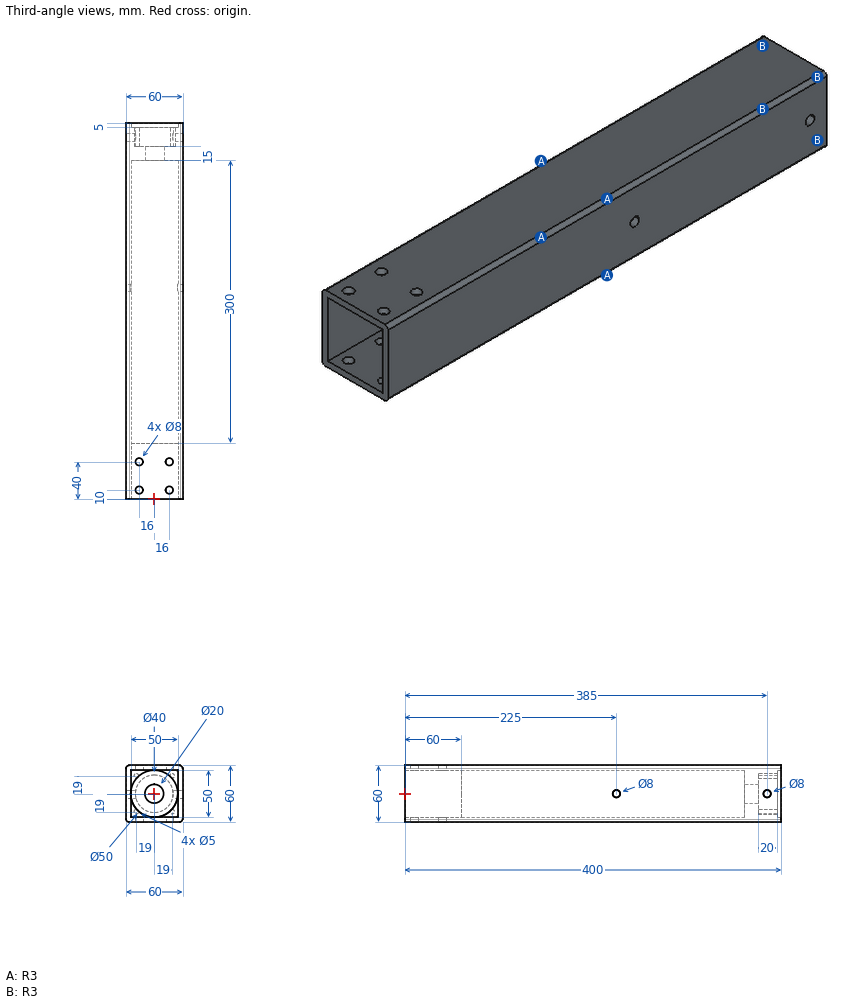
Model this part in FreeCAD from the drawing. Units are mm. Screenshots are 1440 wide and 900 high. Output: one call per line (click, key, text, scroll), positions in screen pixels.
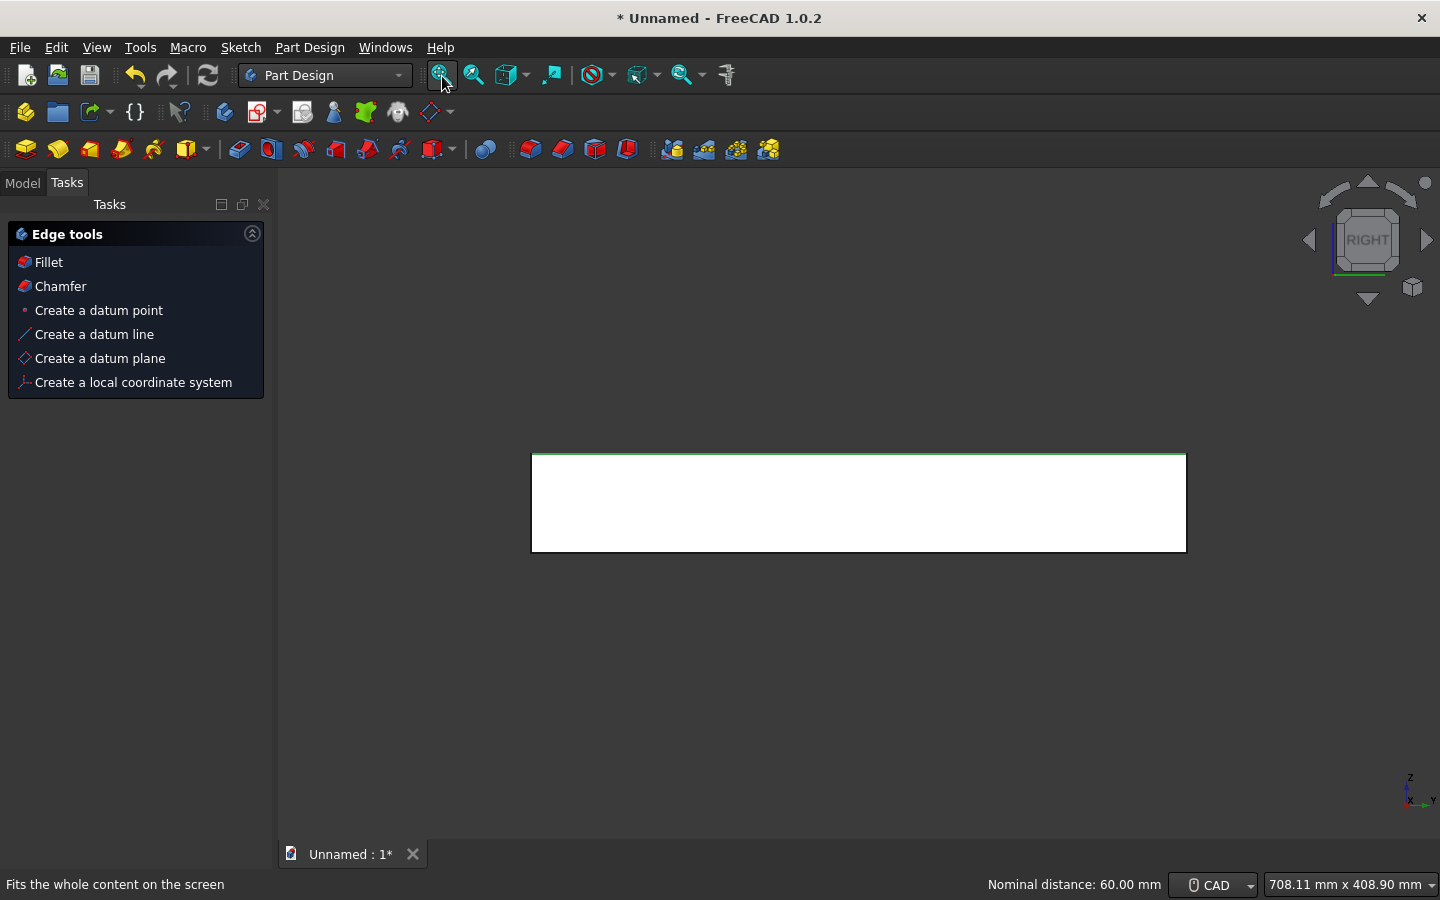
click(859, 552, ctrl)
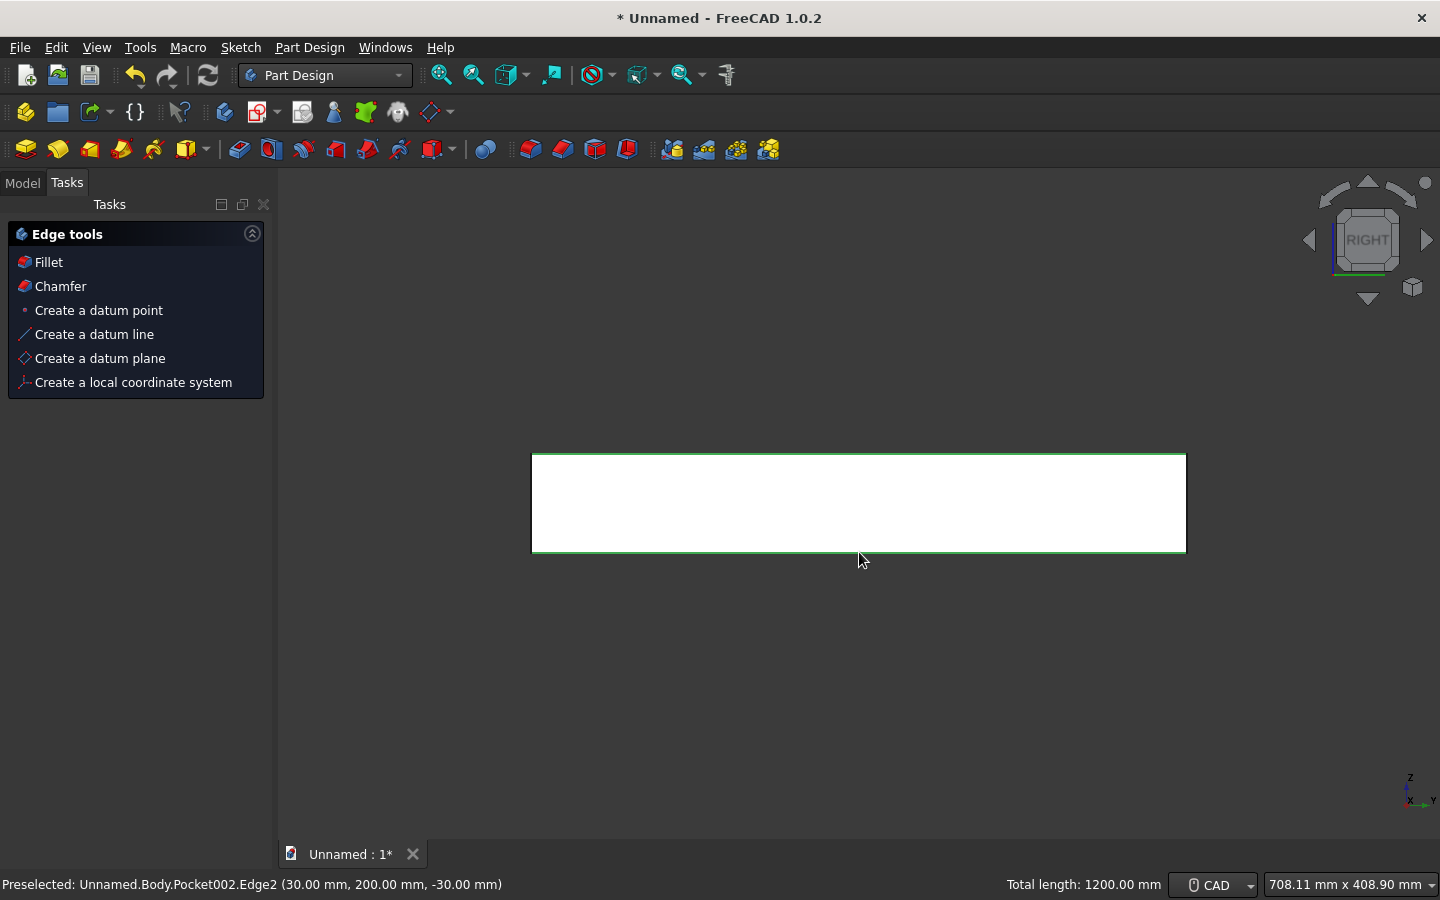
key(5)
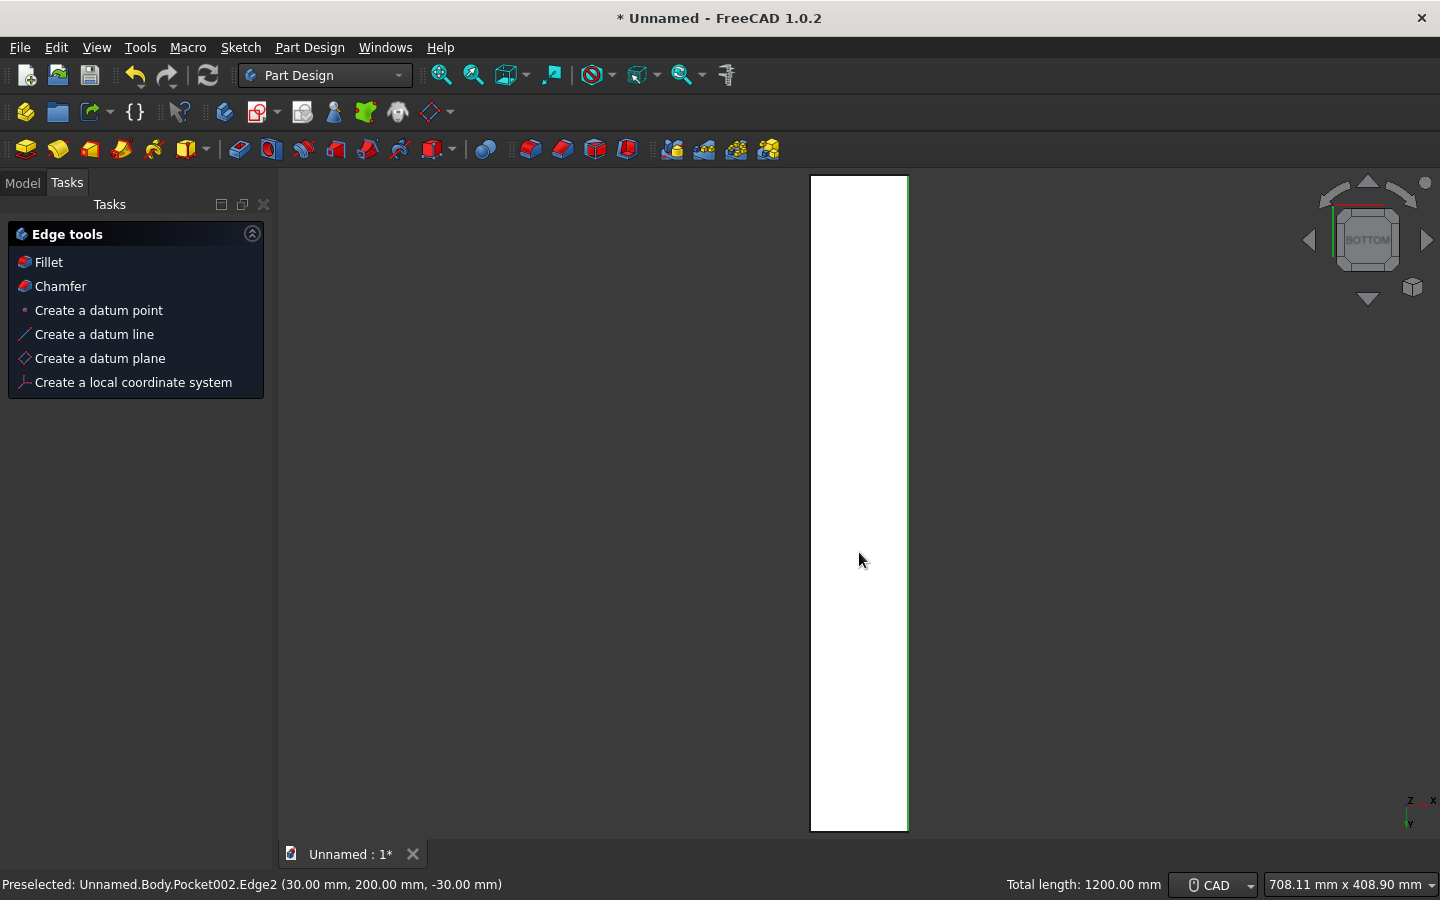
click(810, 502, ctrl)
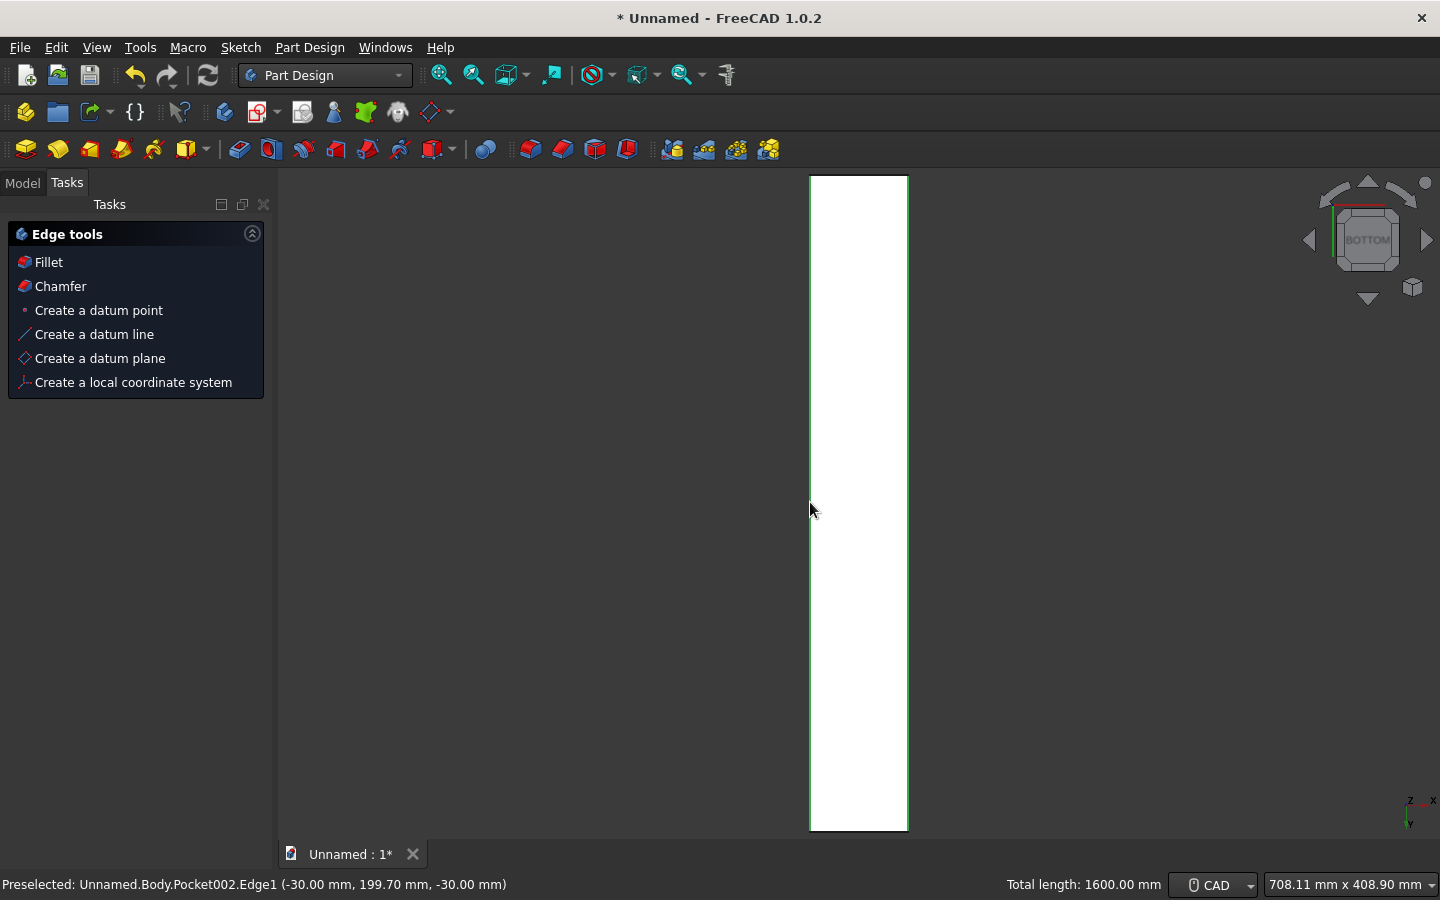
click(532, 150)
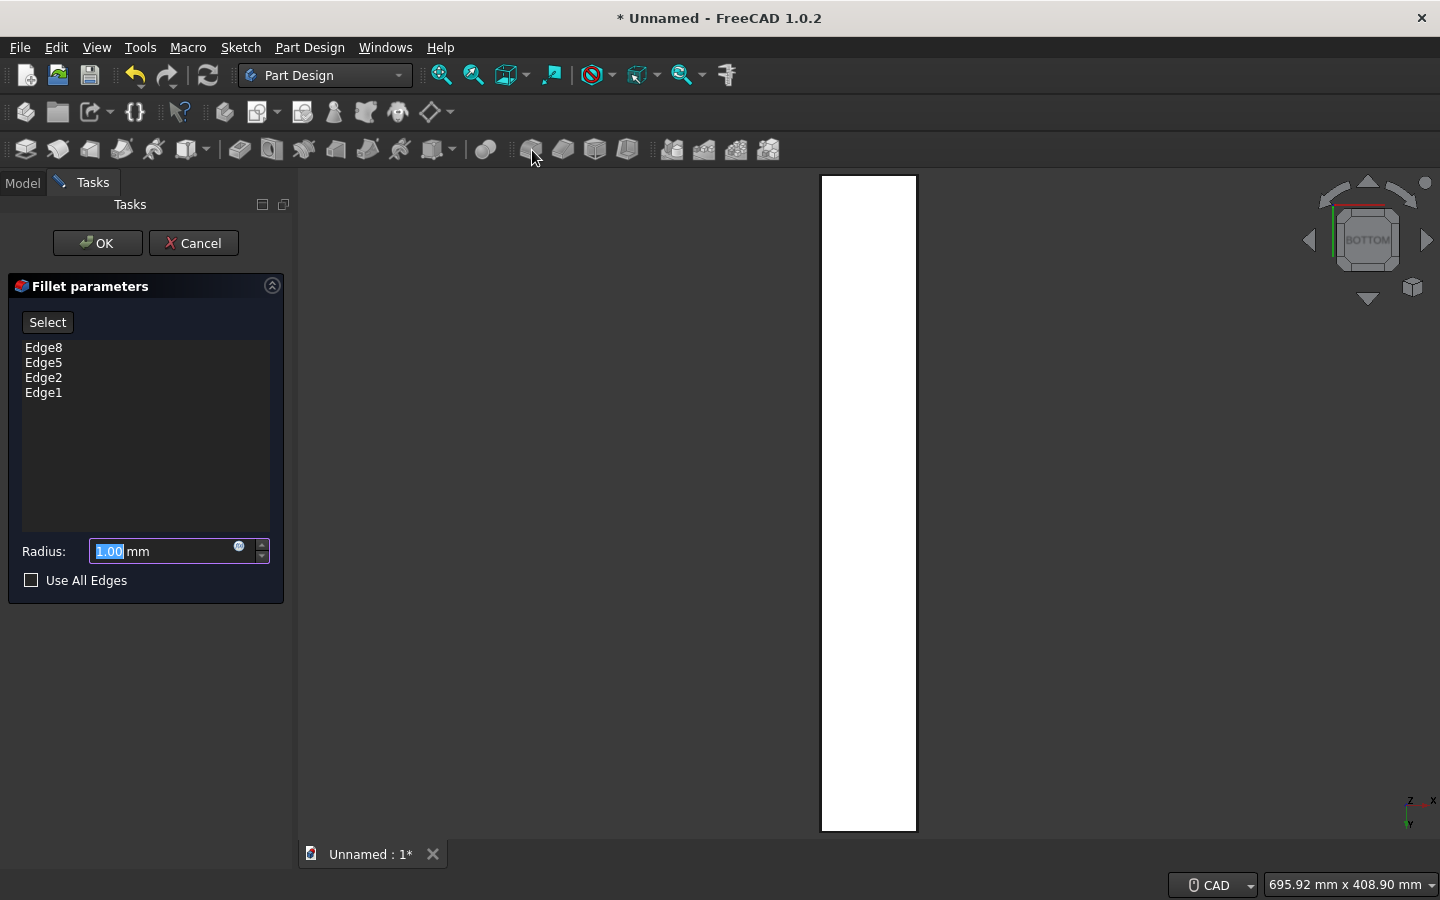
text(3)
key(Tab)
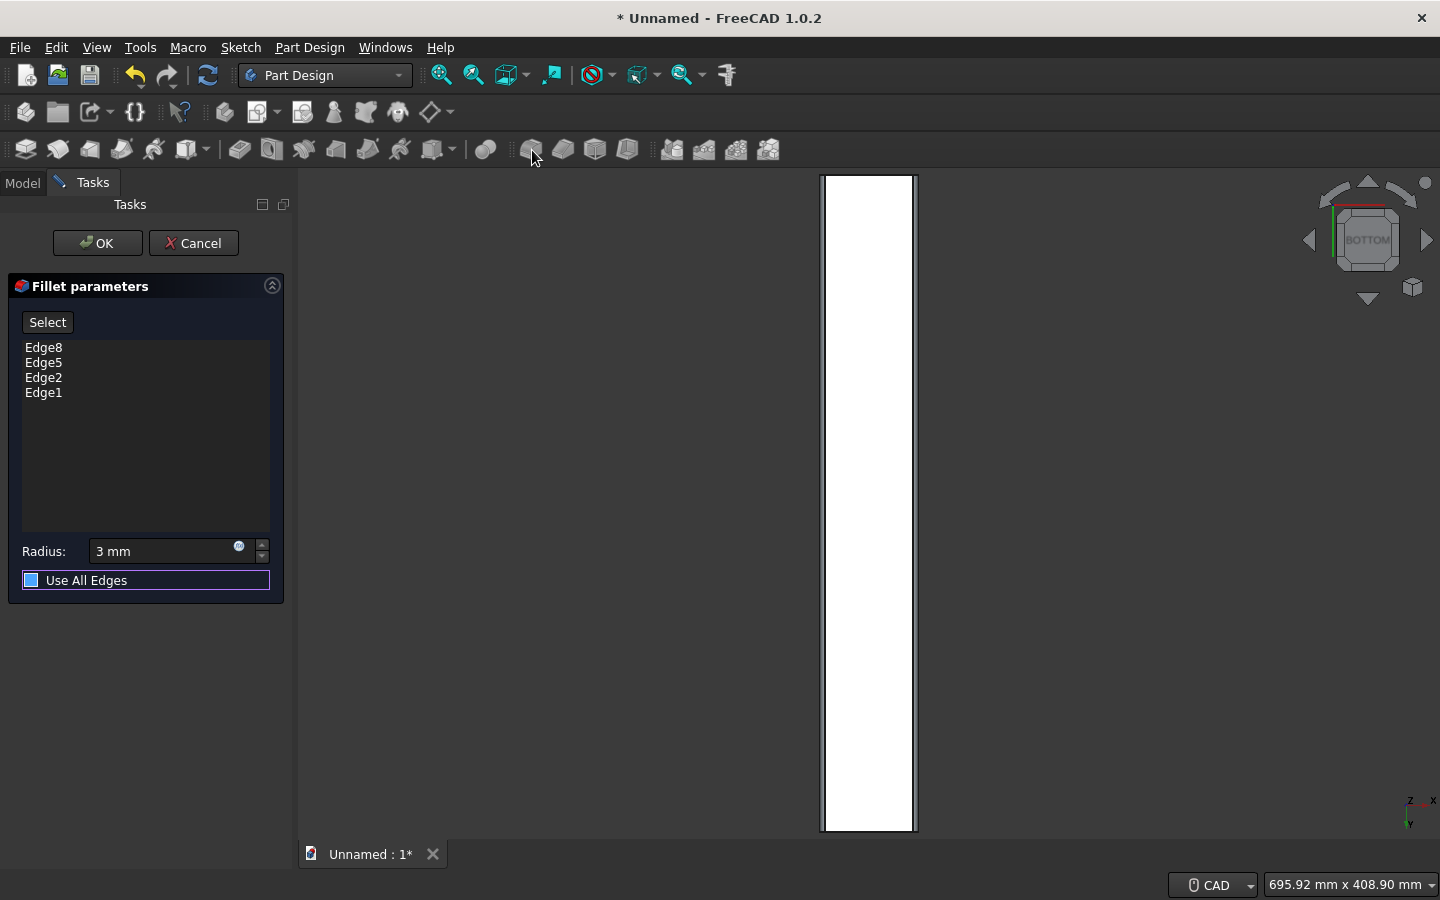
click(98, 243)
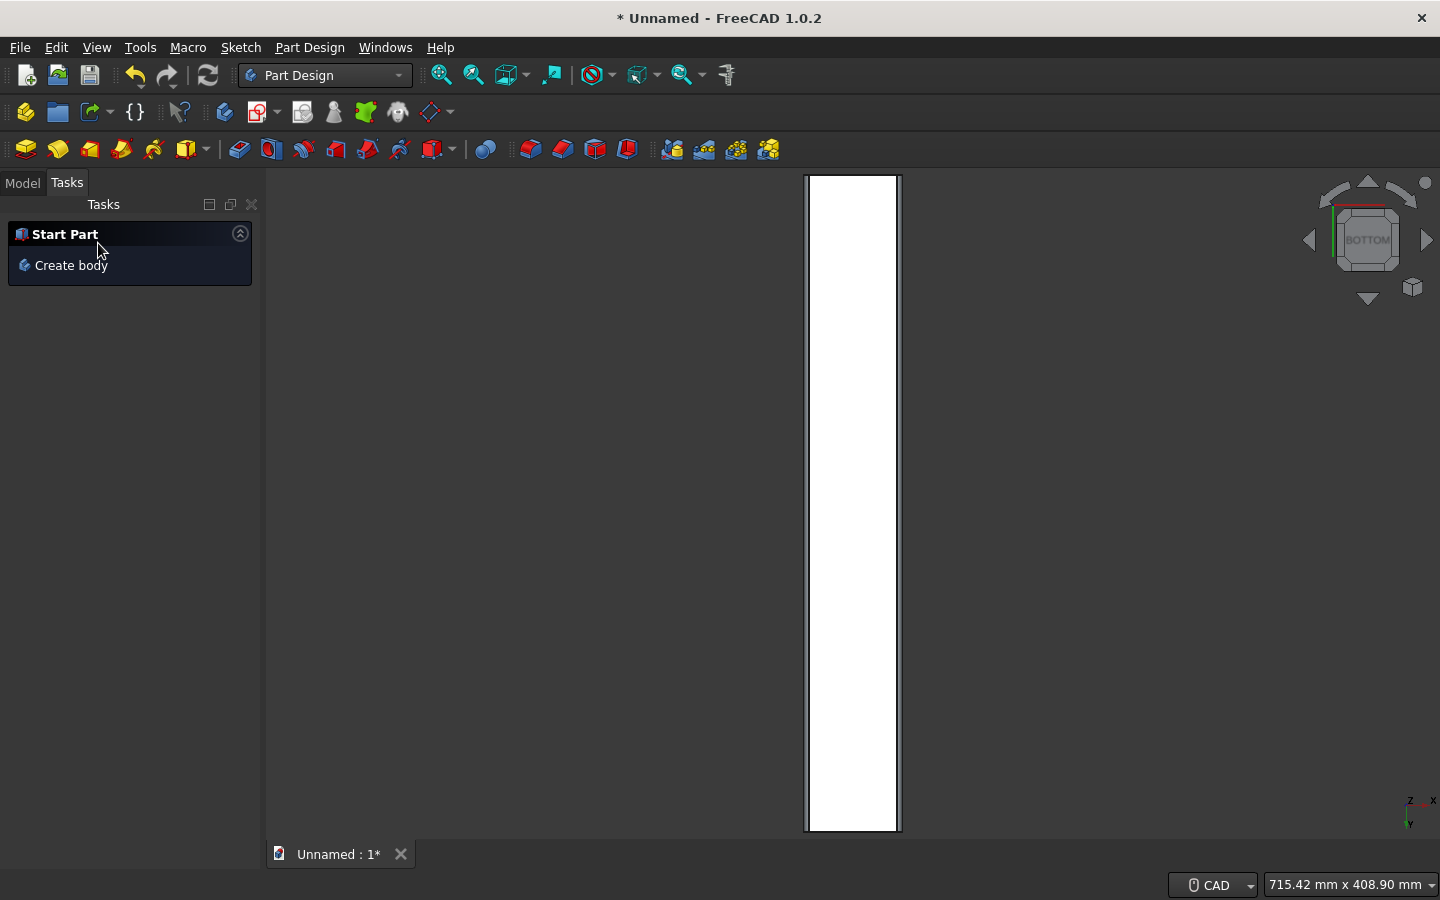
click(258, 112)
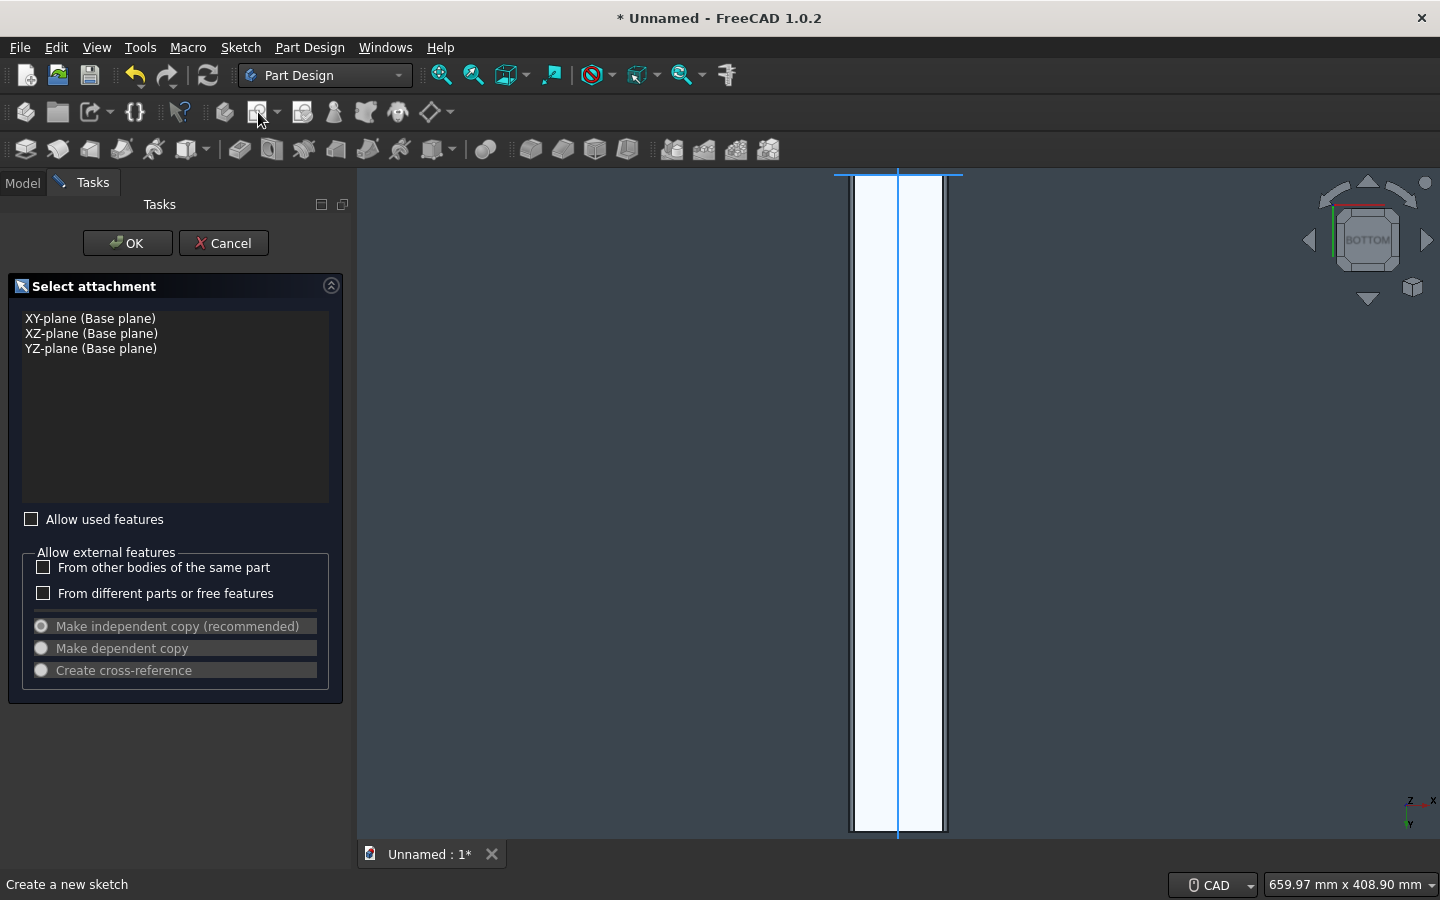
click(82, 348)